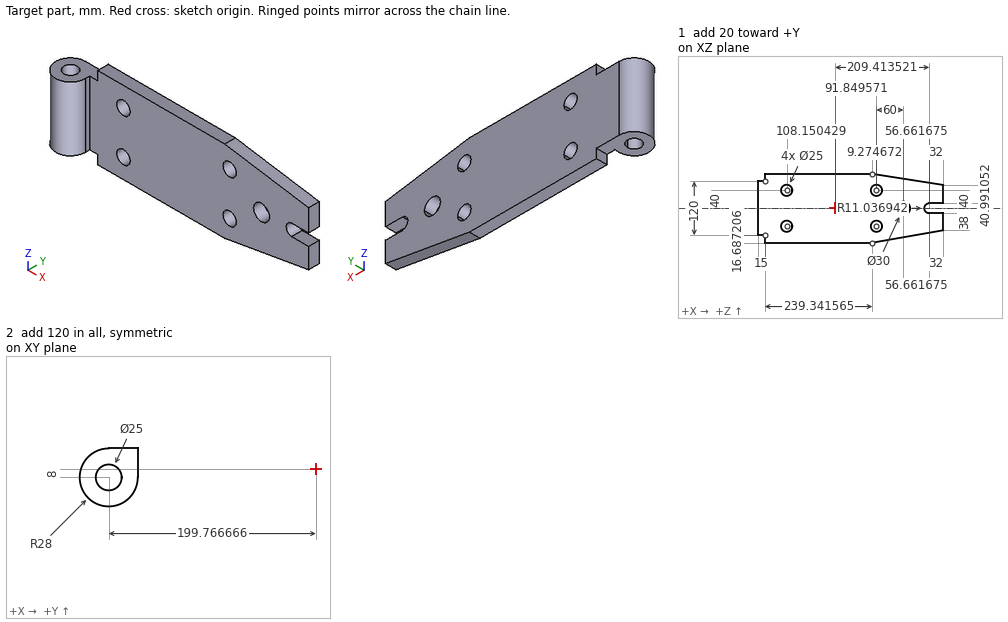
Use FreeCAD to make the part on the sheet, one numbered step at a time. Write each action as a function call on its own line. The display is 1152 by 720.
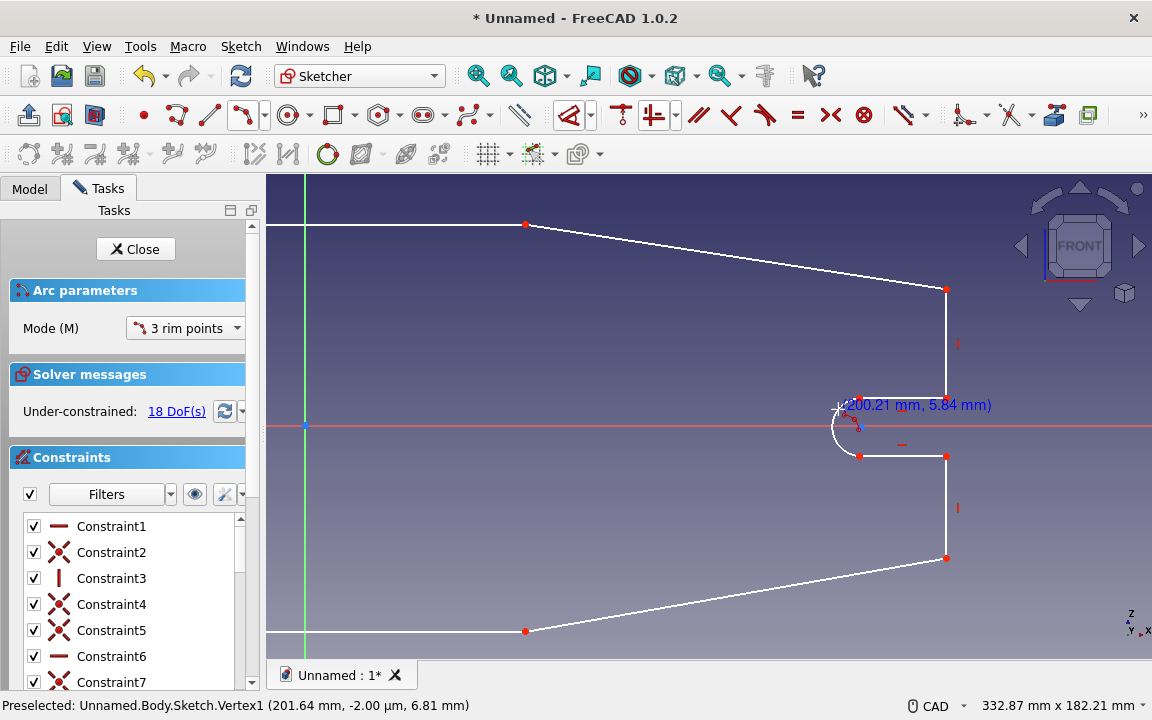
click(288, 116)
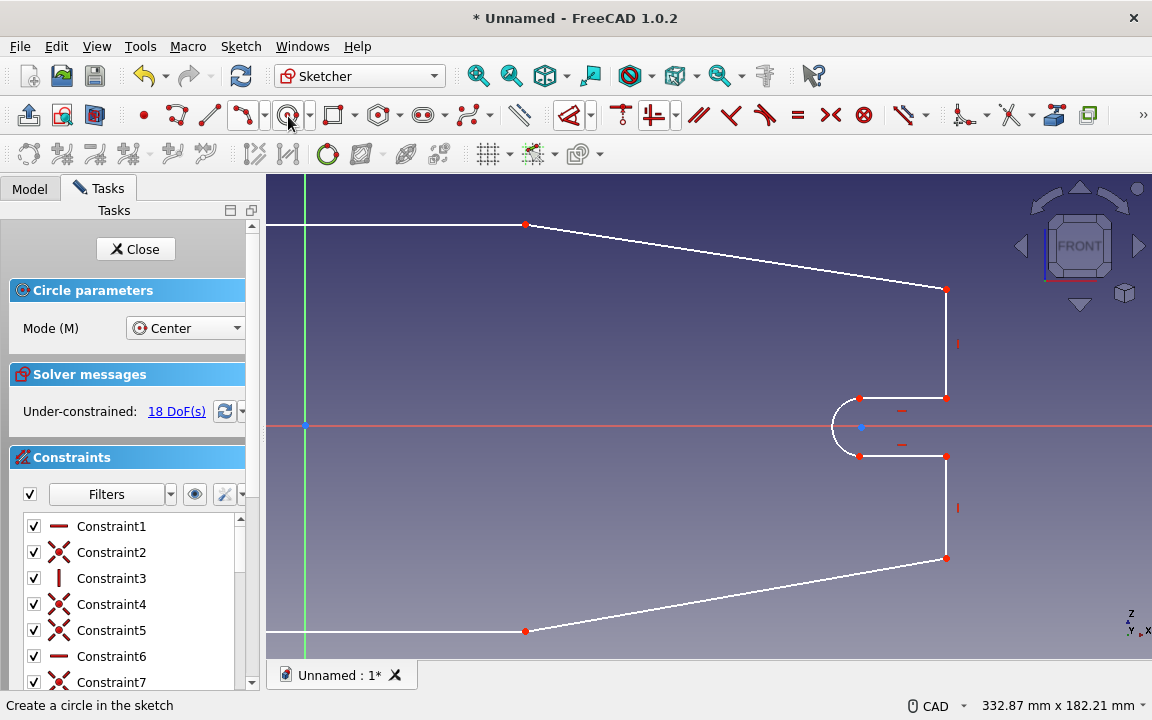
scroll(840, 409, down, 4)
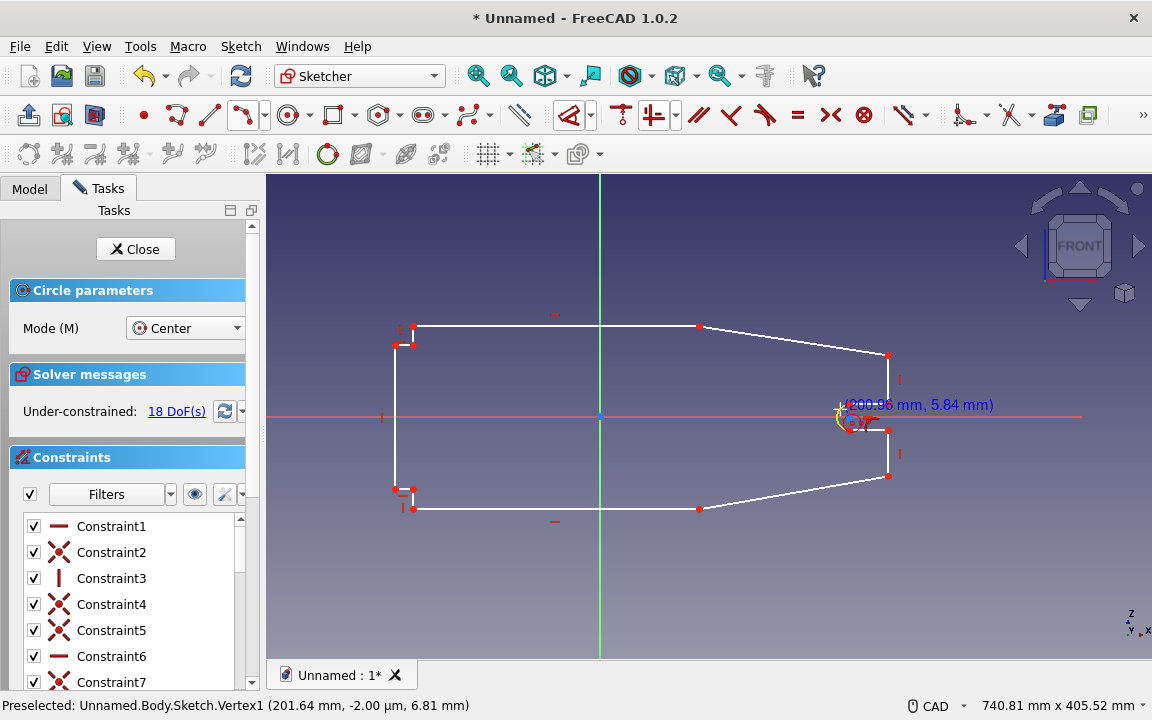
scroll(471, 369, up, 3)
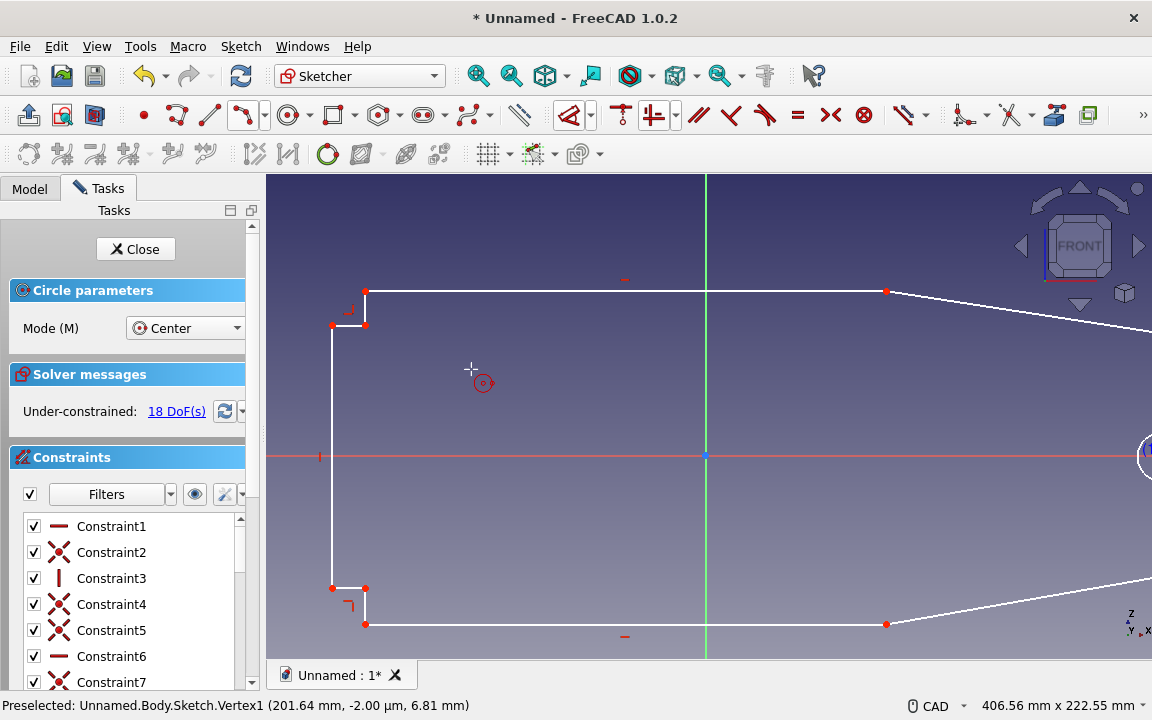
click(470, 368)
click(489, 349)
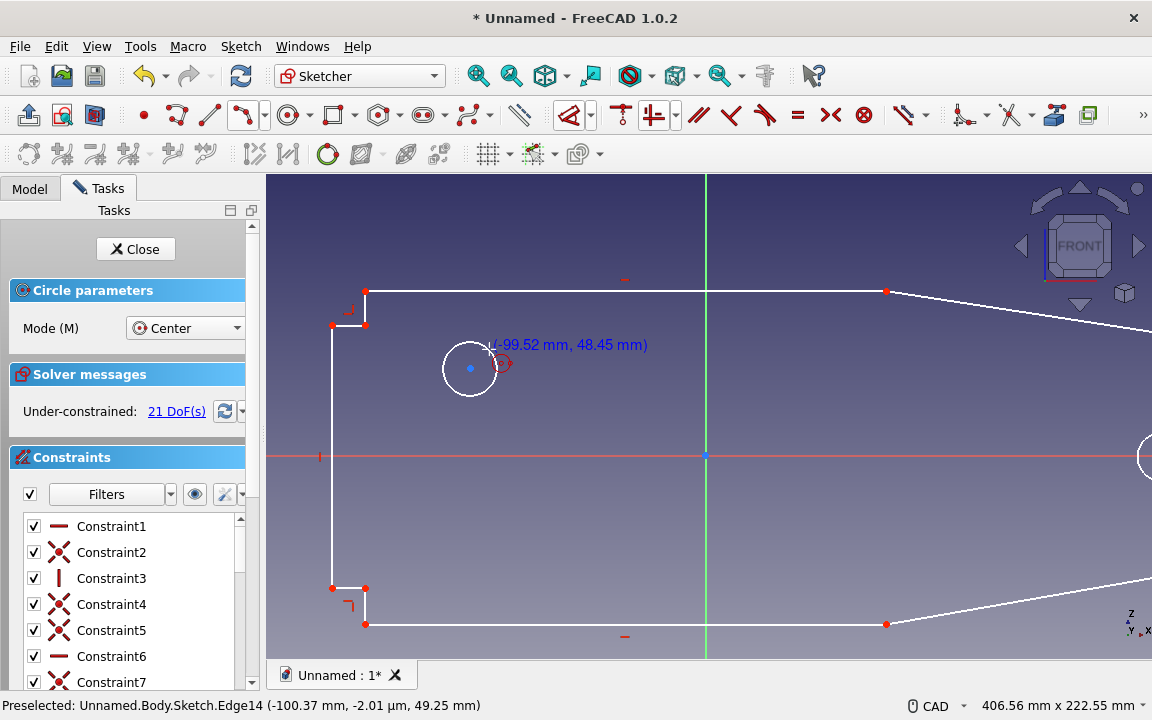
click(906, 368)
click(925, 349)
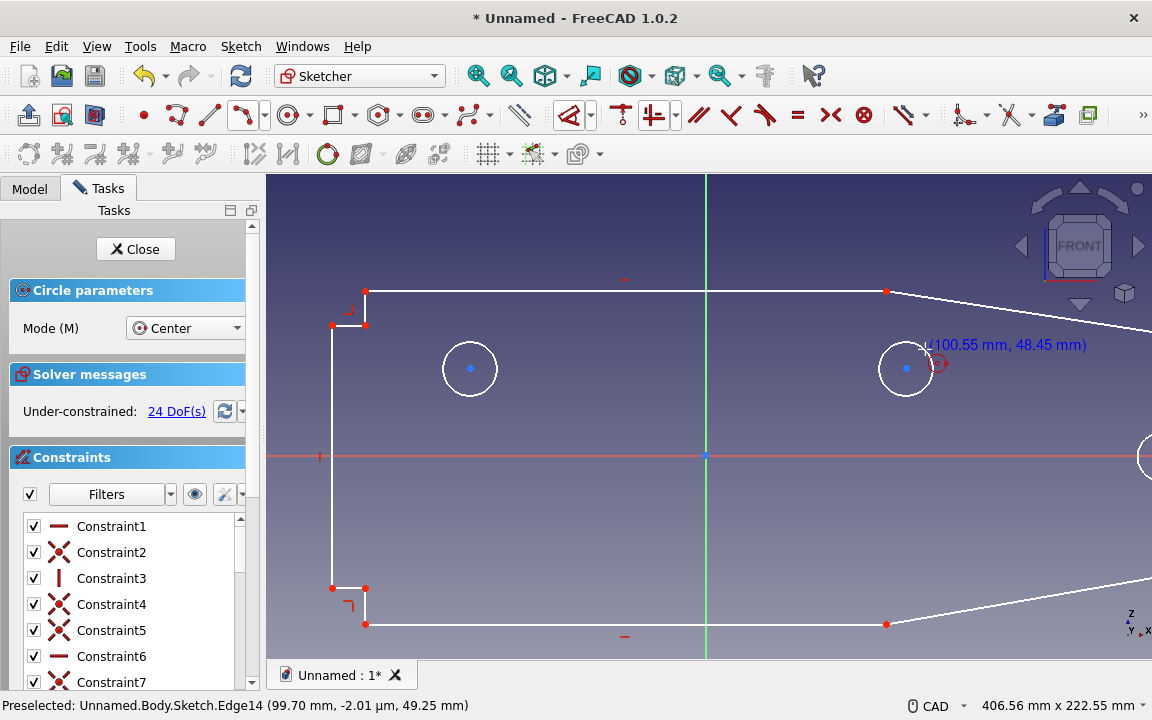
click(470, 543)
click(489, 523)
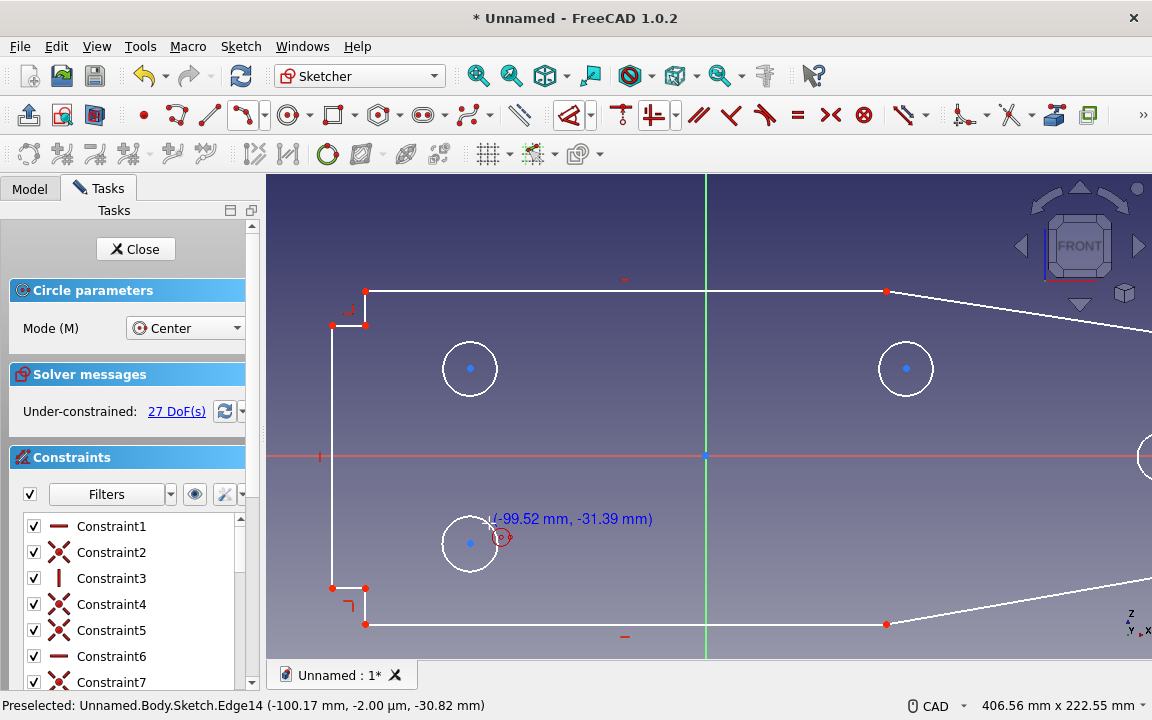
scroll(470, 369, down, 3)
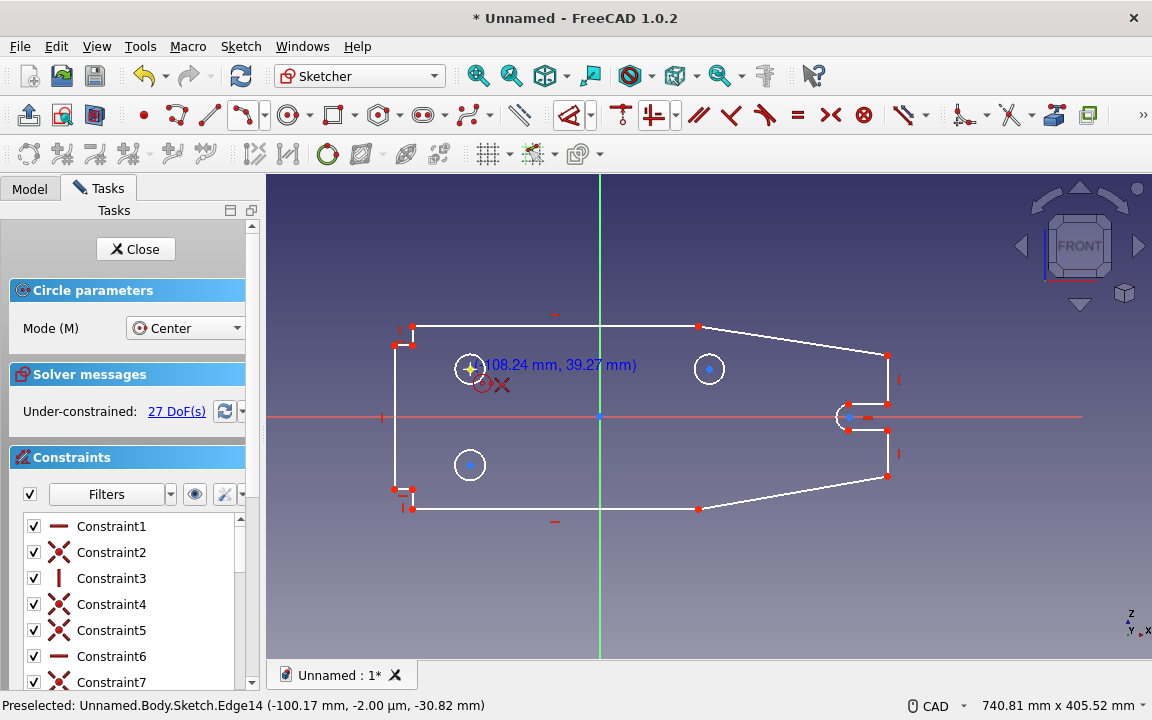
scroll(781, 417, up, 2)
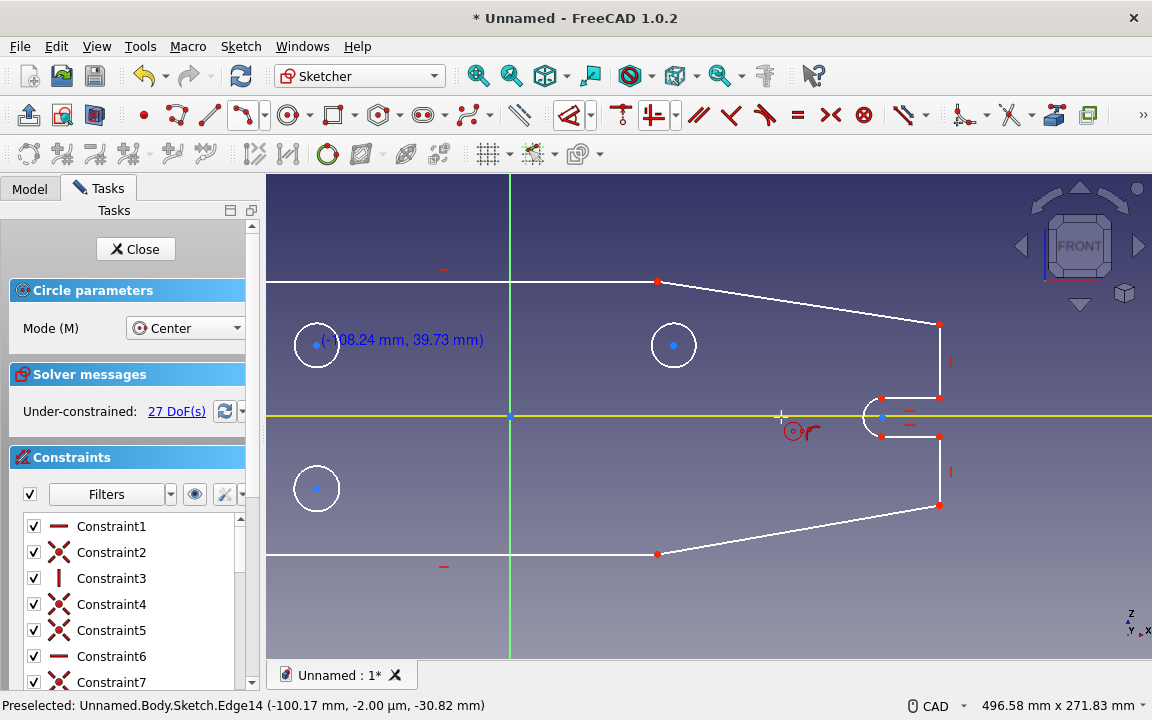
click(781, 416)
click(800, 397)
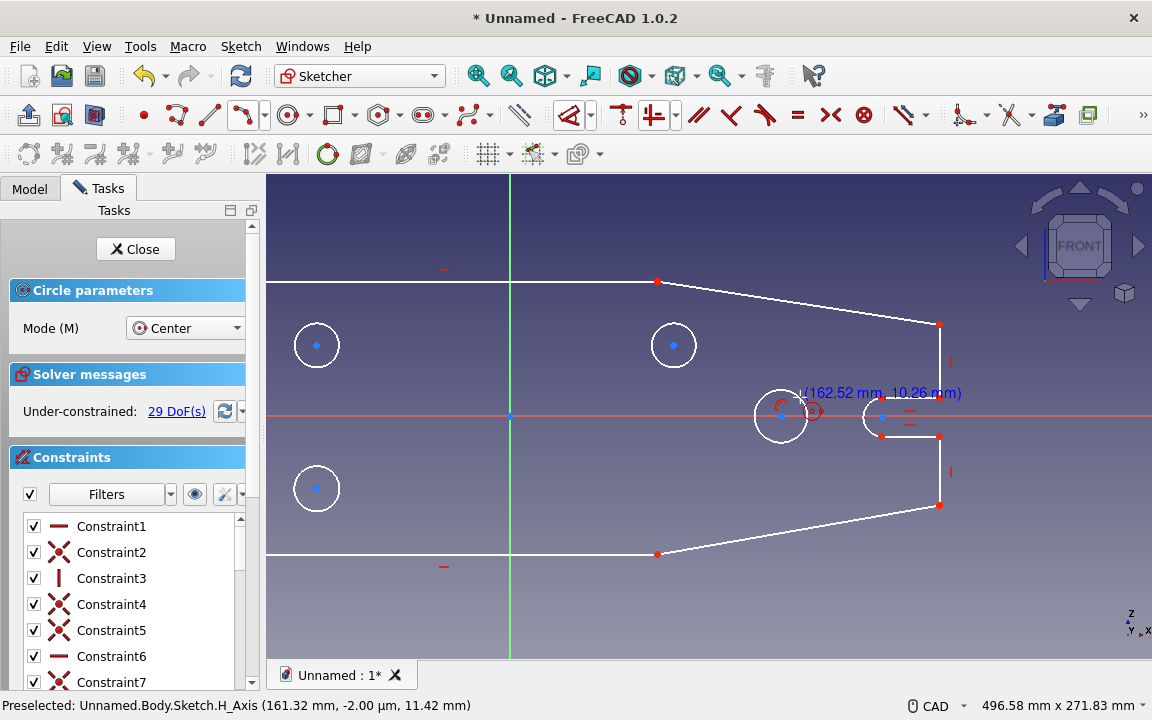
click(674, 488)
click(690, 472)
key(Escape)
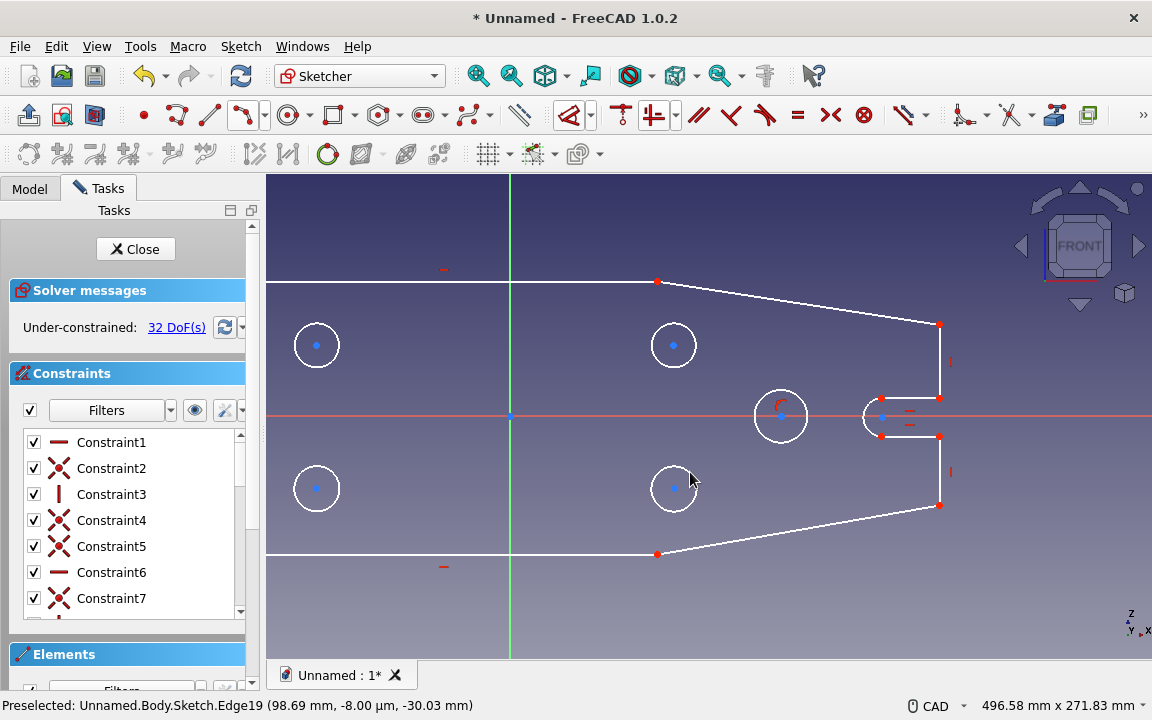
click(332, 330)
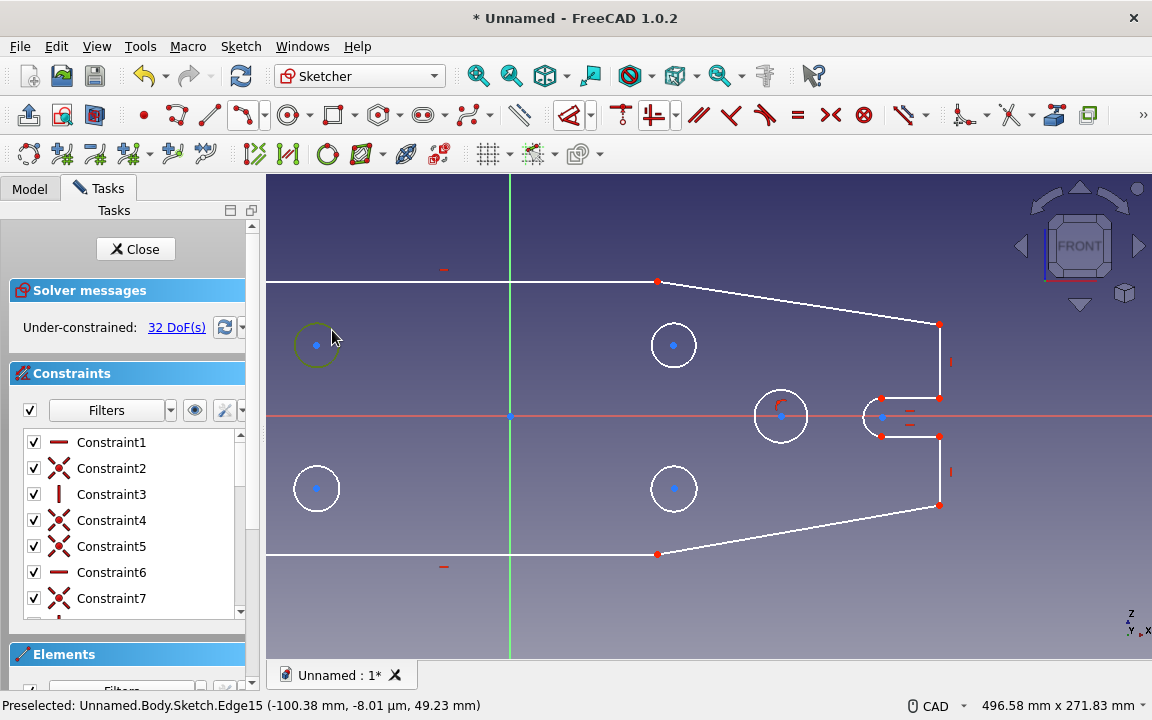
click(689, 330)